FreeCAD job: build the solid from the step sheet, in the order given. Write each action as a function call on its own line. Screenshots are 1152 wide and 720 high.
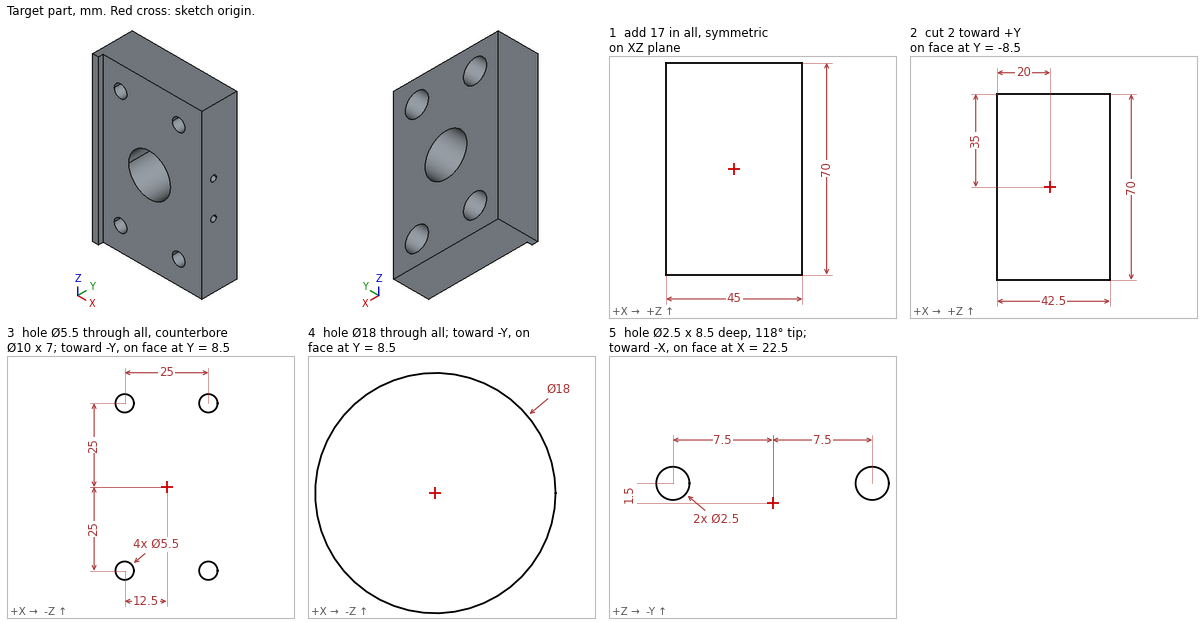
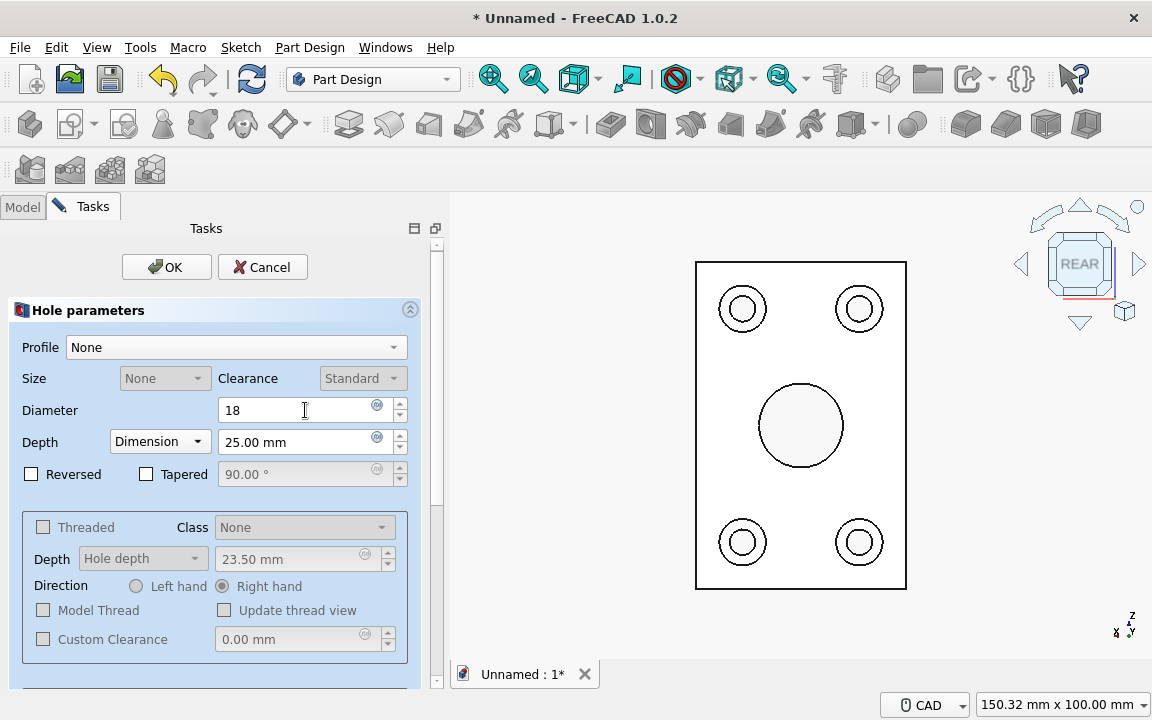
click(161, 442)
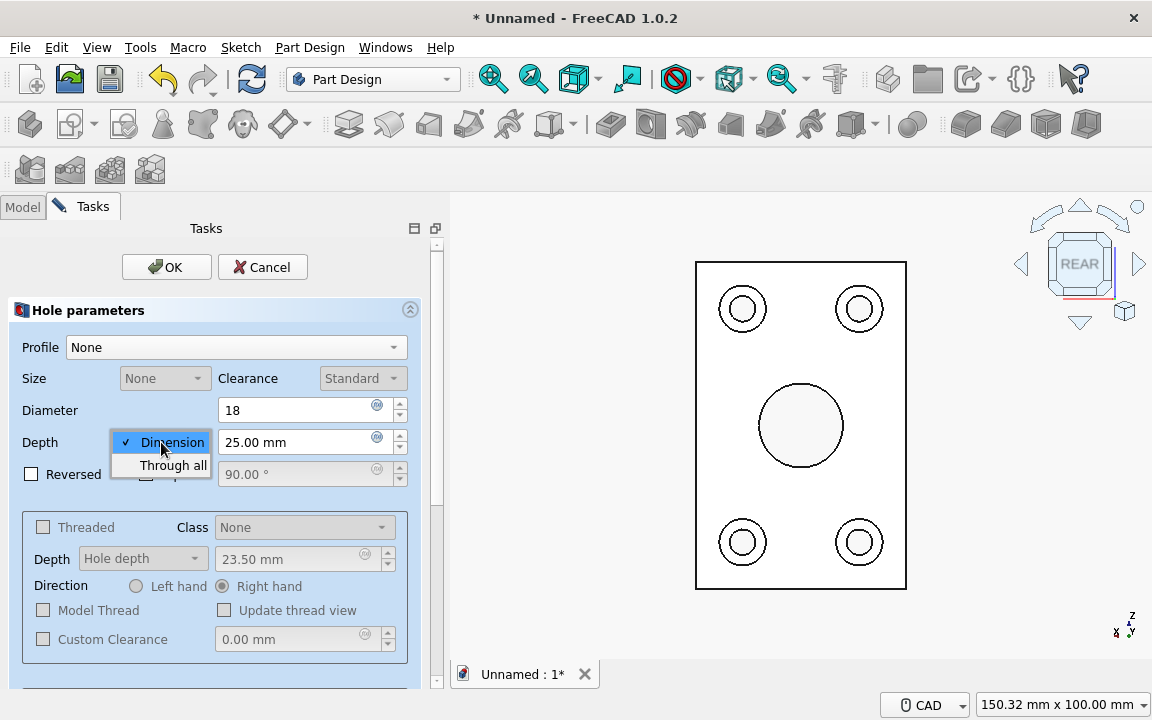
click(160, 466)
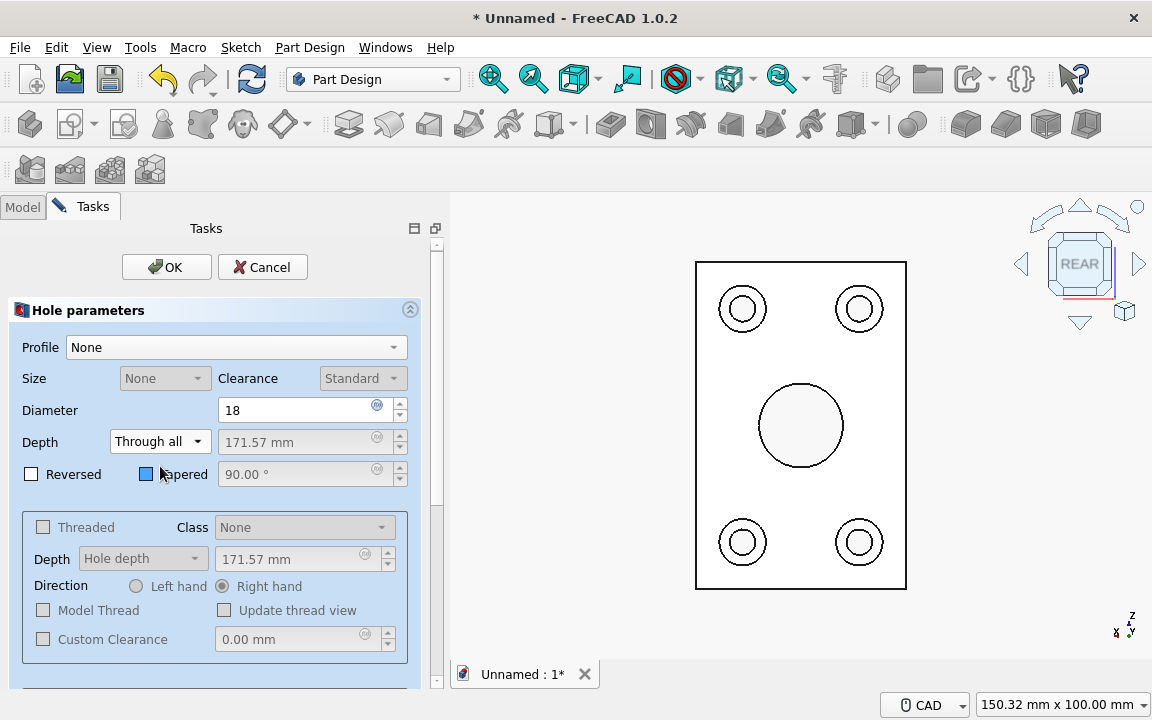
click(167, 267)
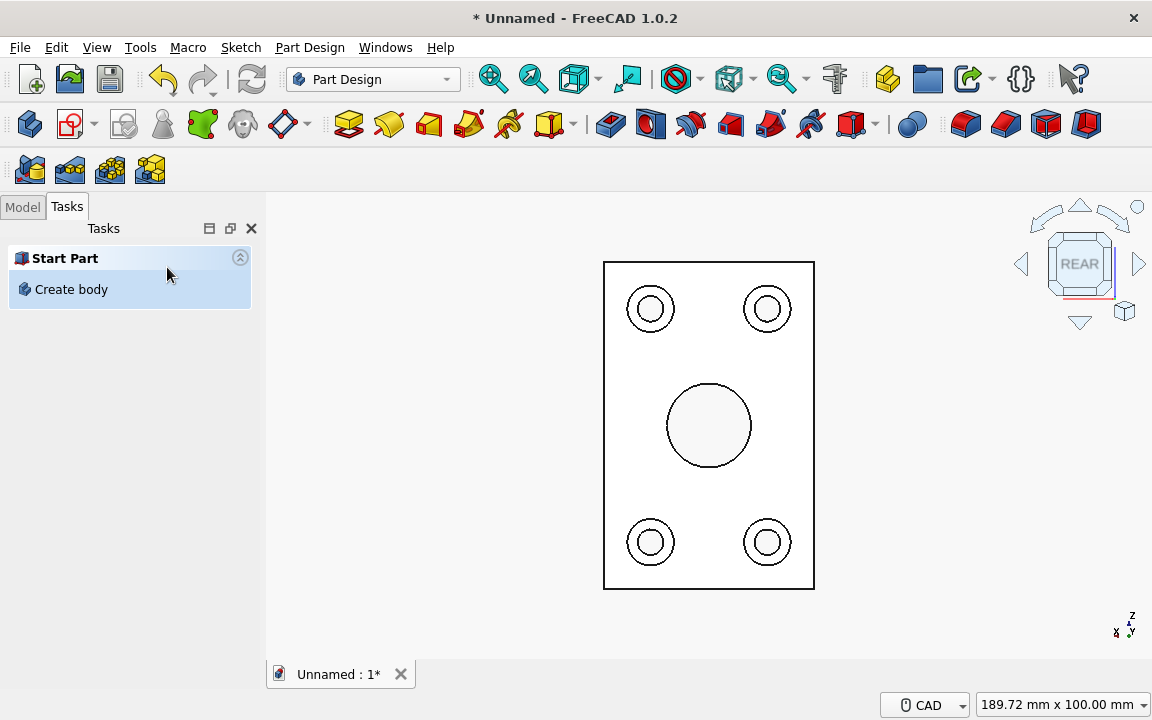
key(0)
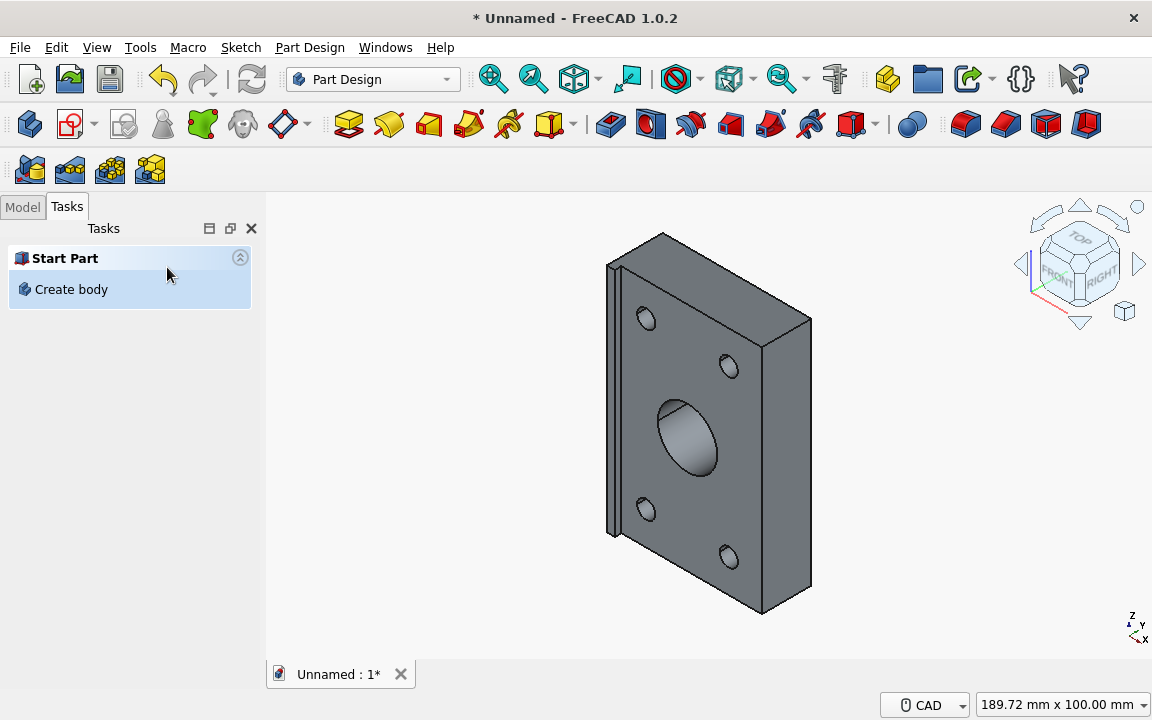
click(787, 427)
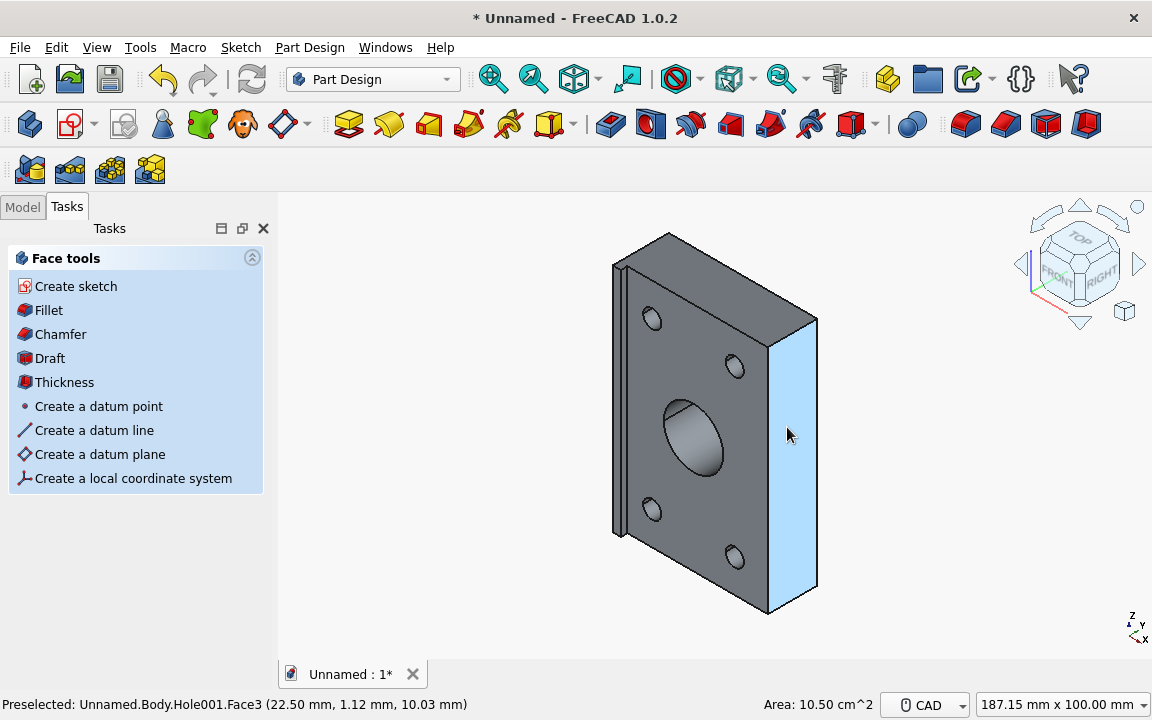
click(70, 124)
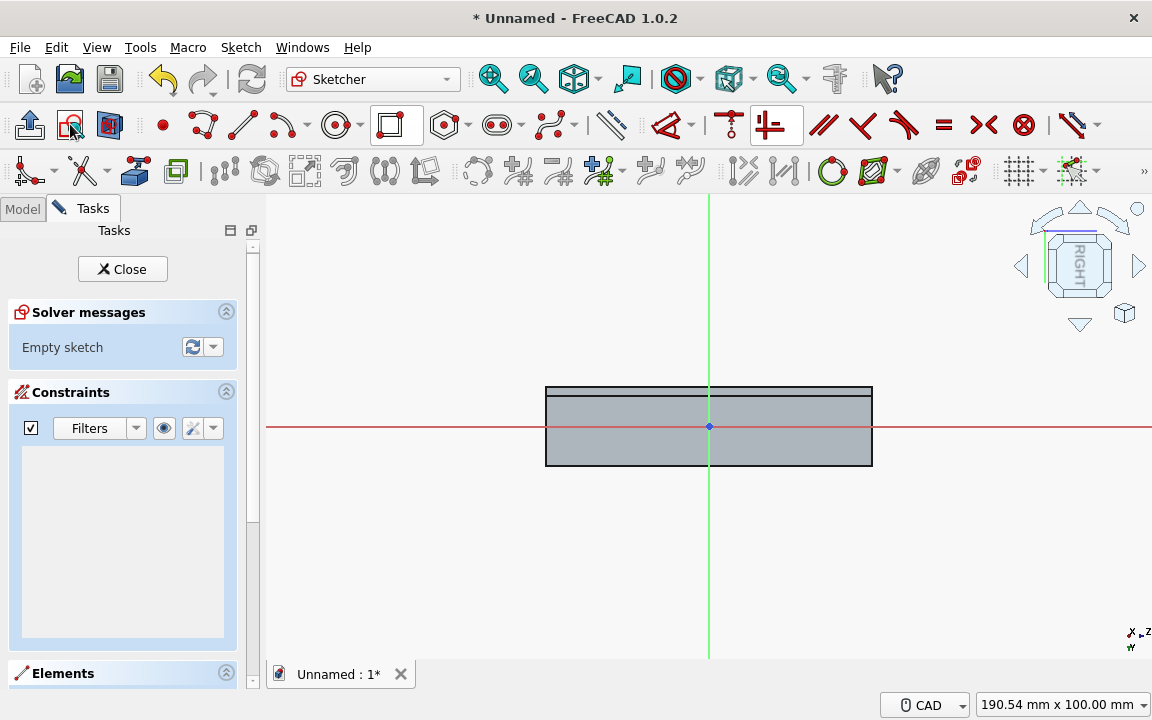
scroll(723, 419, up, 9)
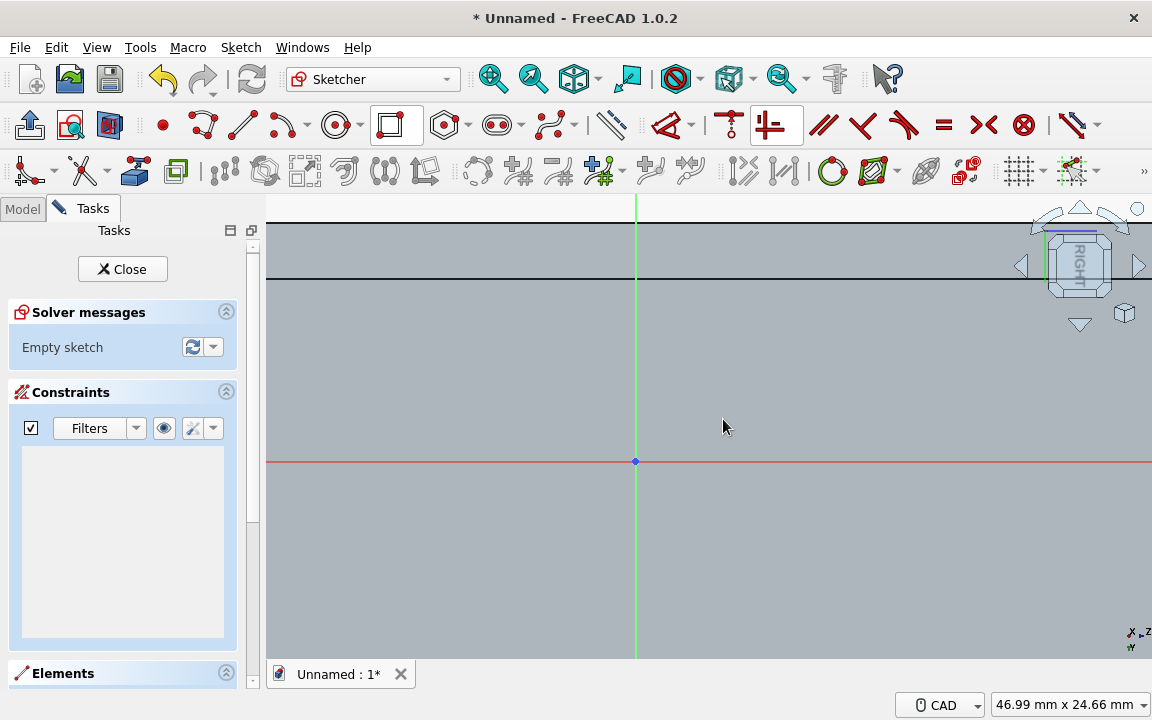
click(336, 126)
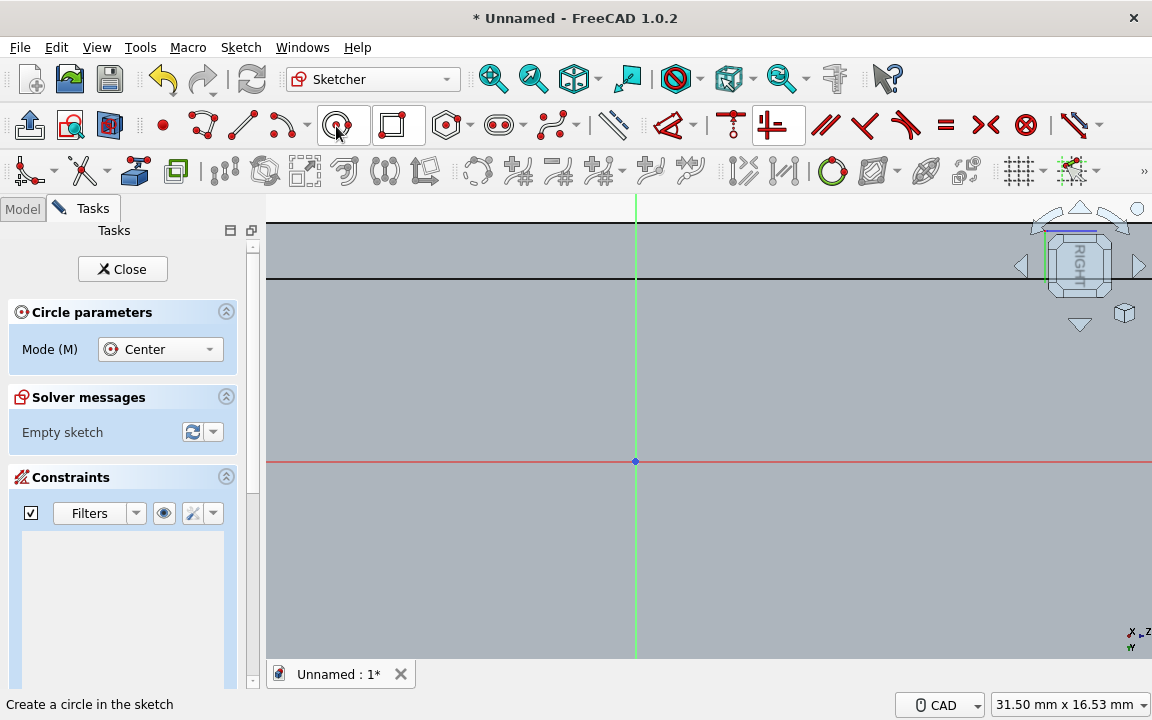
click(425, 420)
move(450, 395)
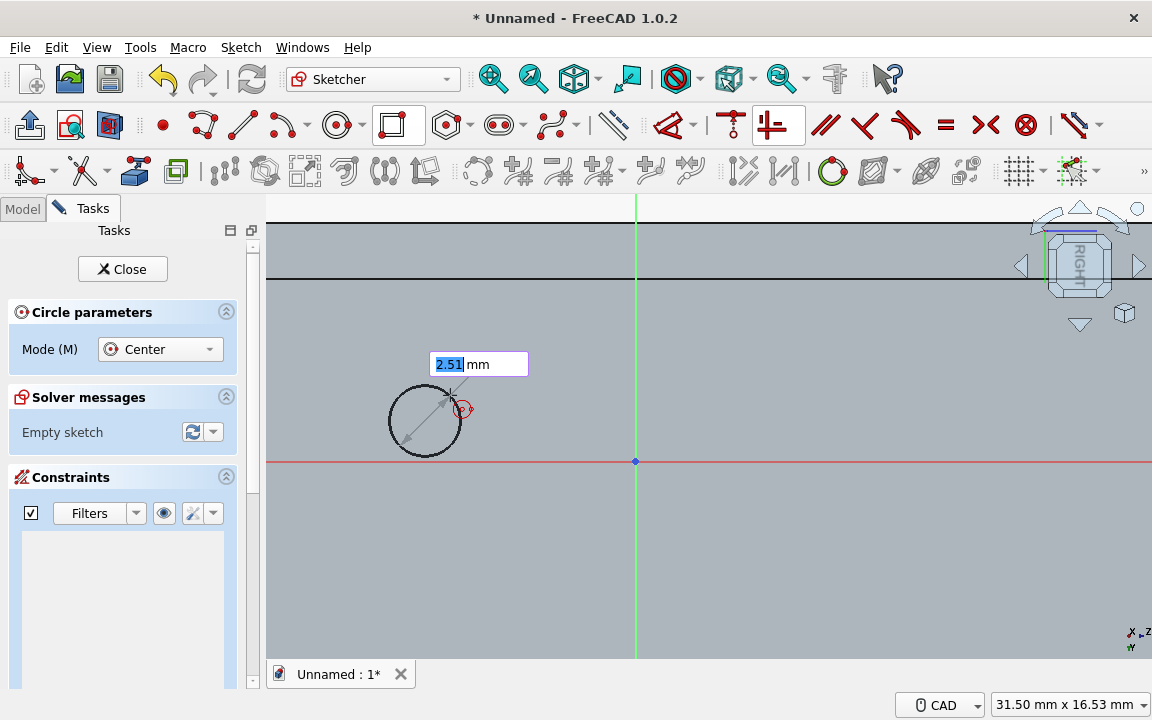
text(2.5)
key(Return)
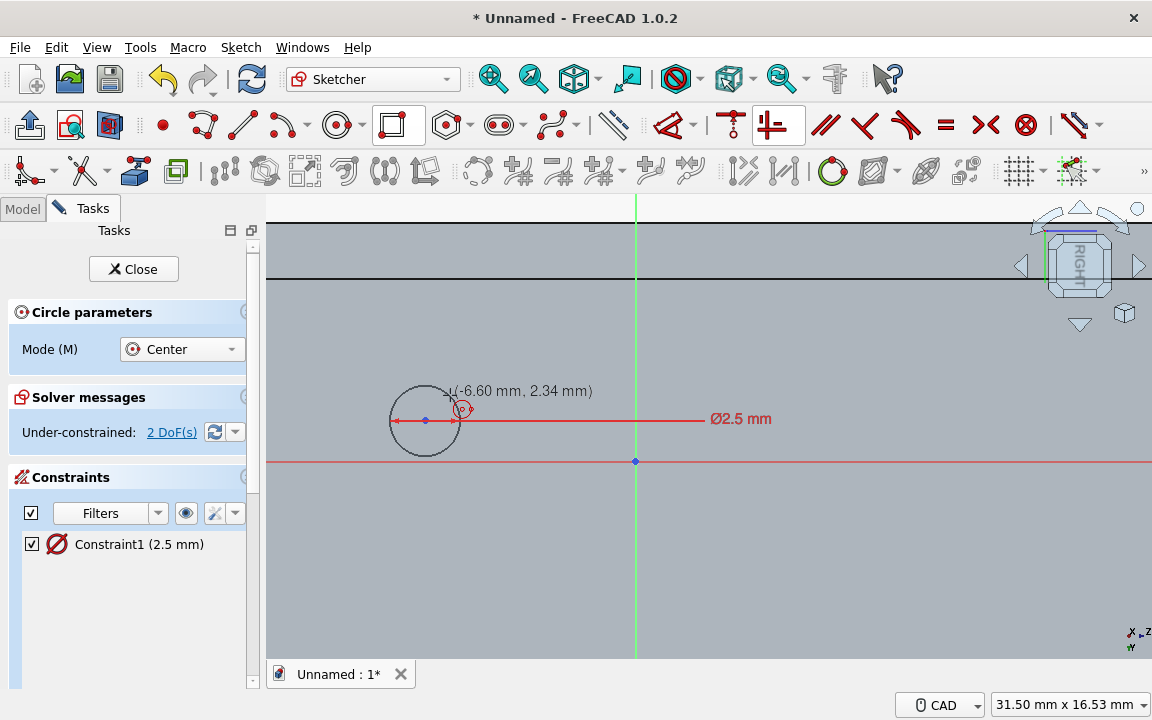
click(847, 420)
move(872, 395)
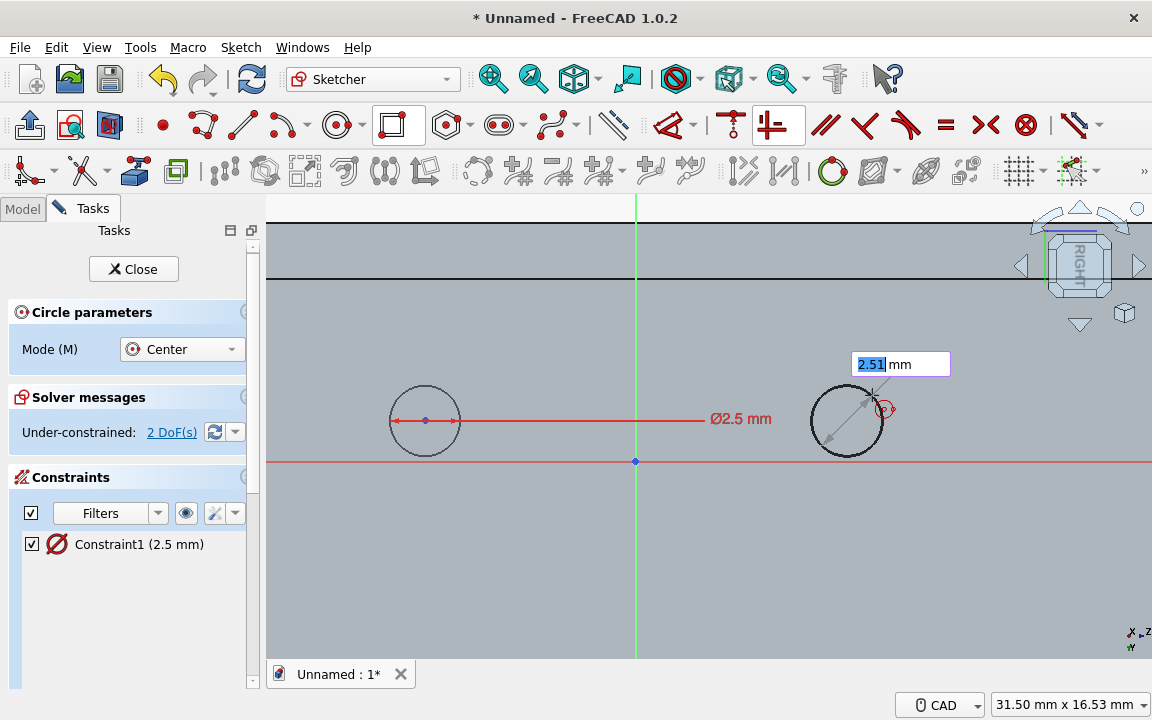
text(2.5)
key(Return)
key(Escape)